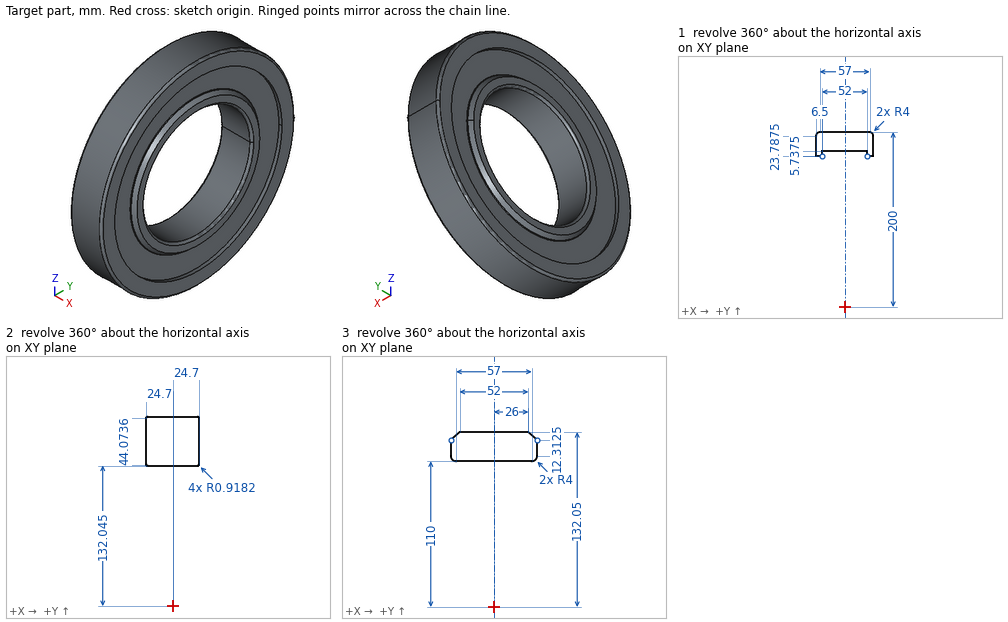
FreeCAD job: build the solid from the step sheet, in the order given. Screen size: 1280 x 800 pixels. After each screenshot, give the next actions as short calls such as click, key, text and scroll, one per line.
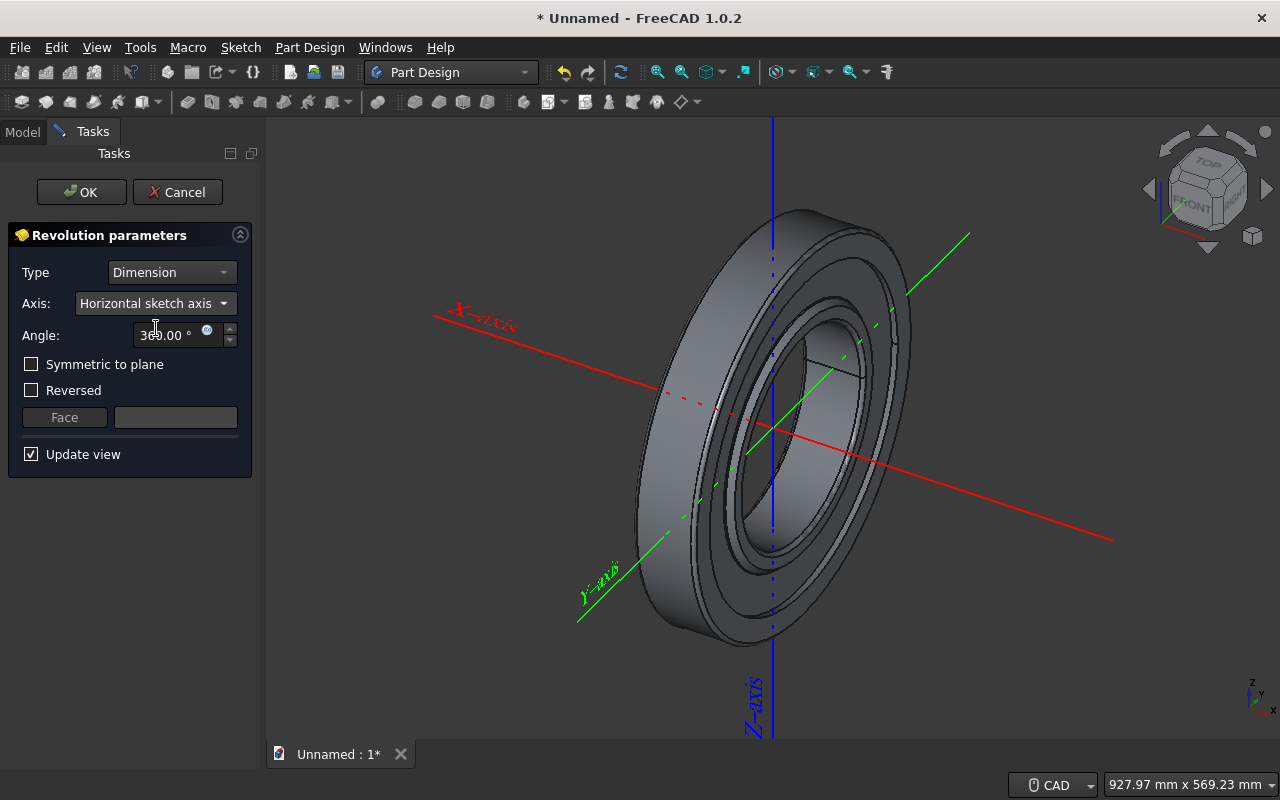
click(82, 192)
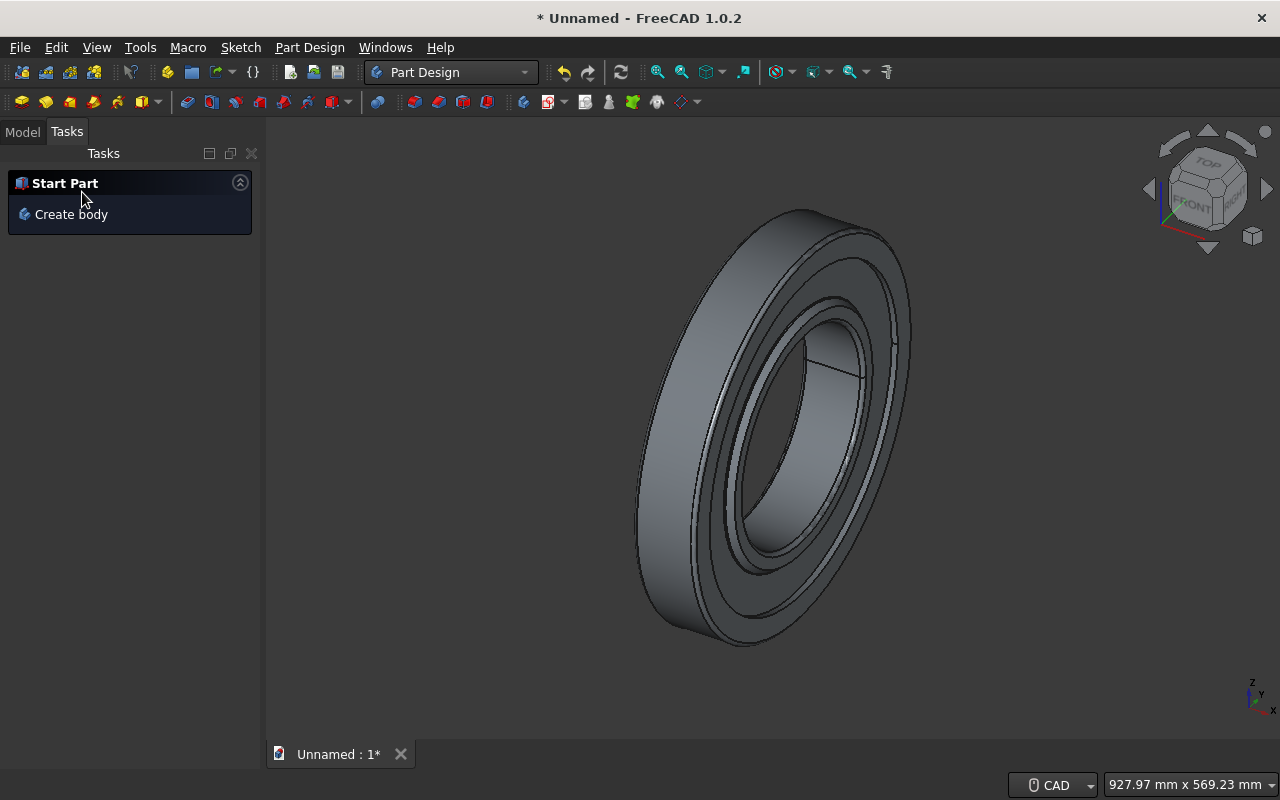
key(0)